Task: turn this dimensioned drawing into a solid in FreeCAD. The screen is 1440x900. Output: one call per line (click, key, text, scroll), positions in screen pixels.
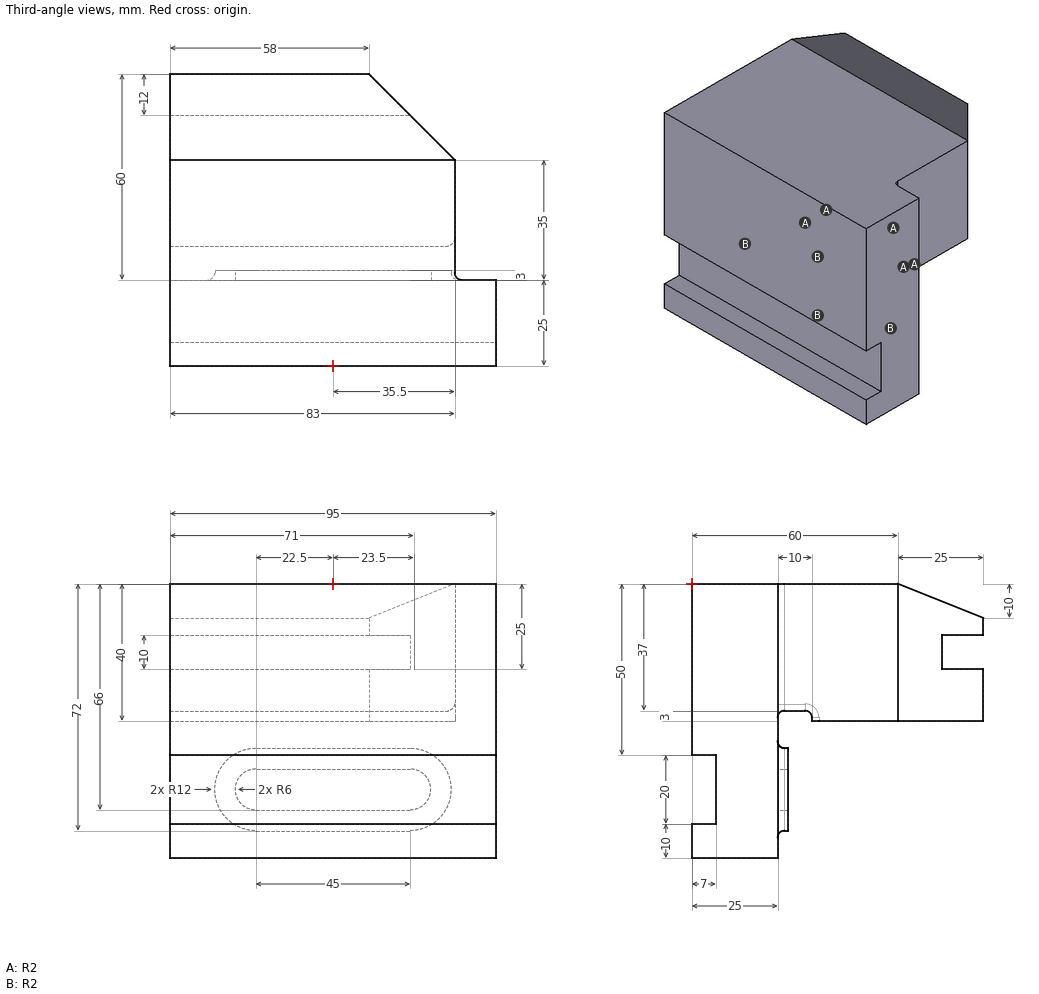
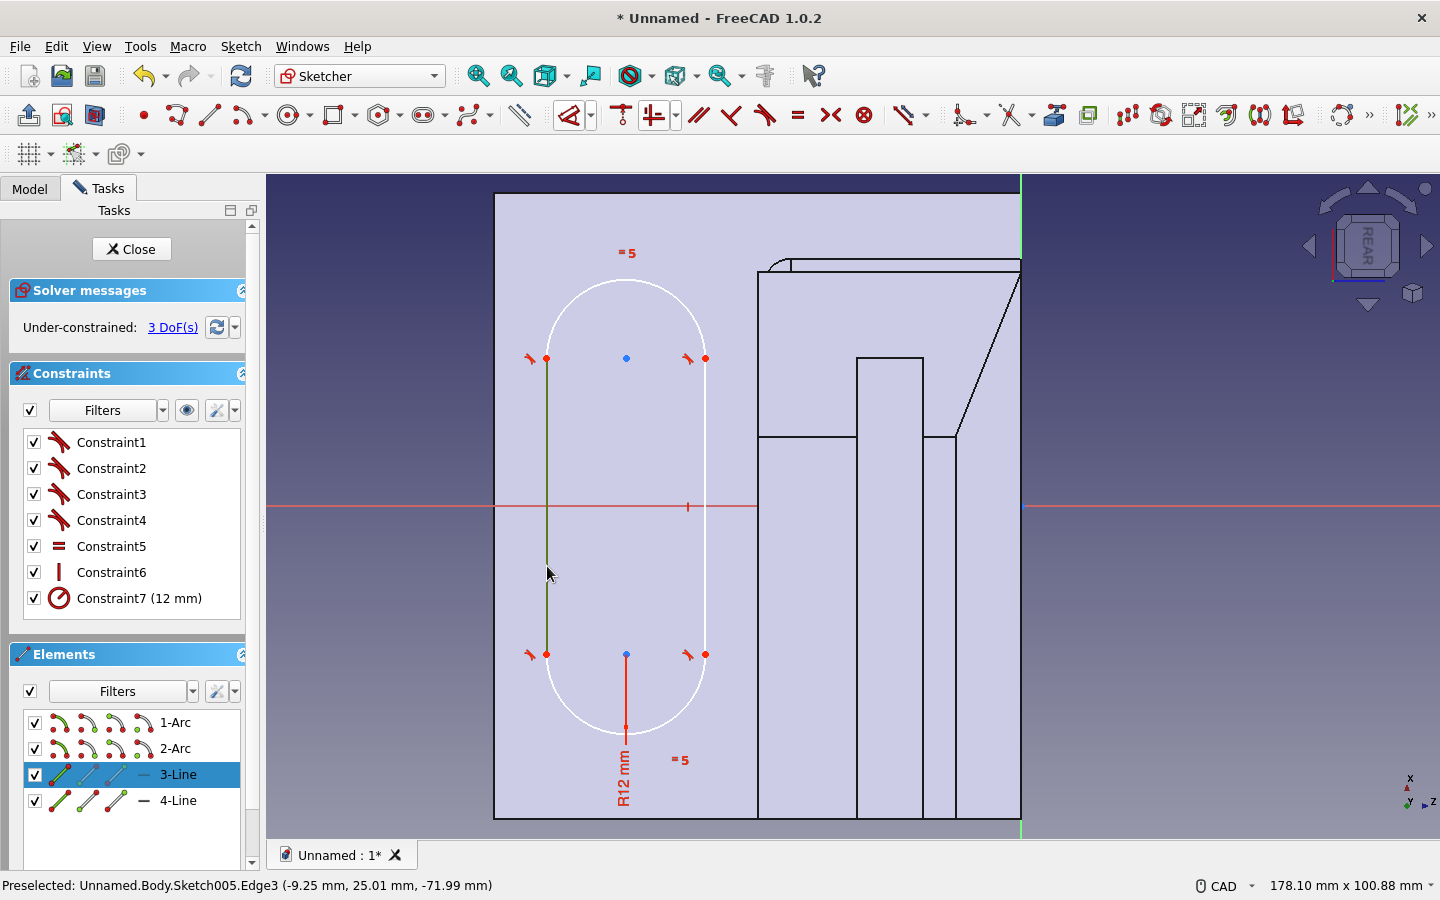
click(590, 116)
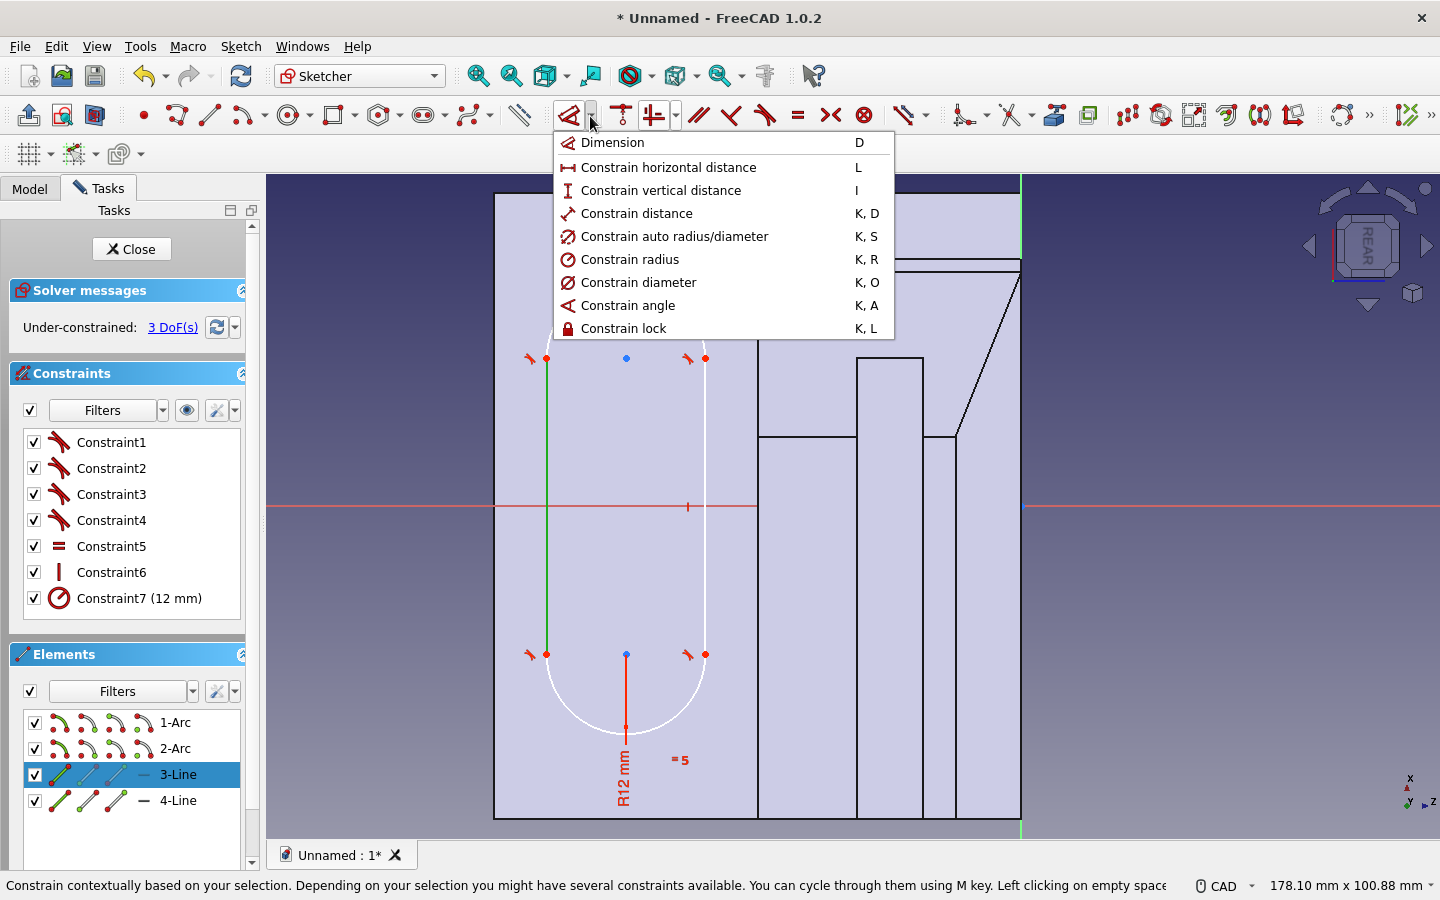
click(724, 190)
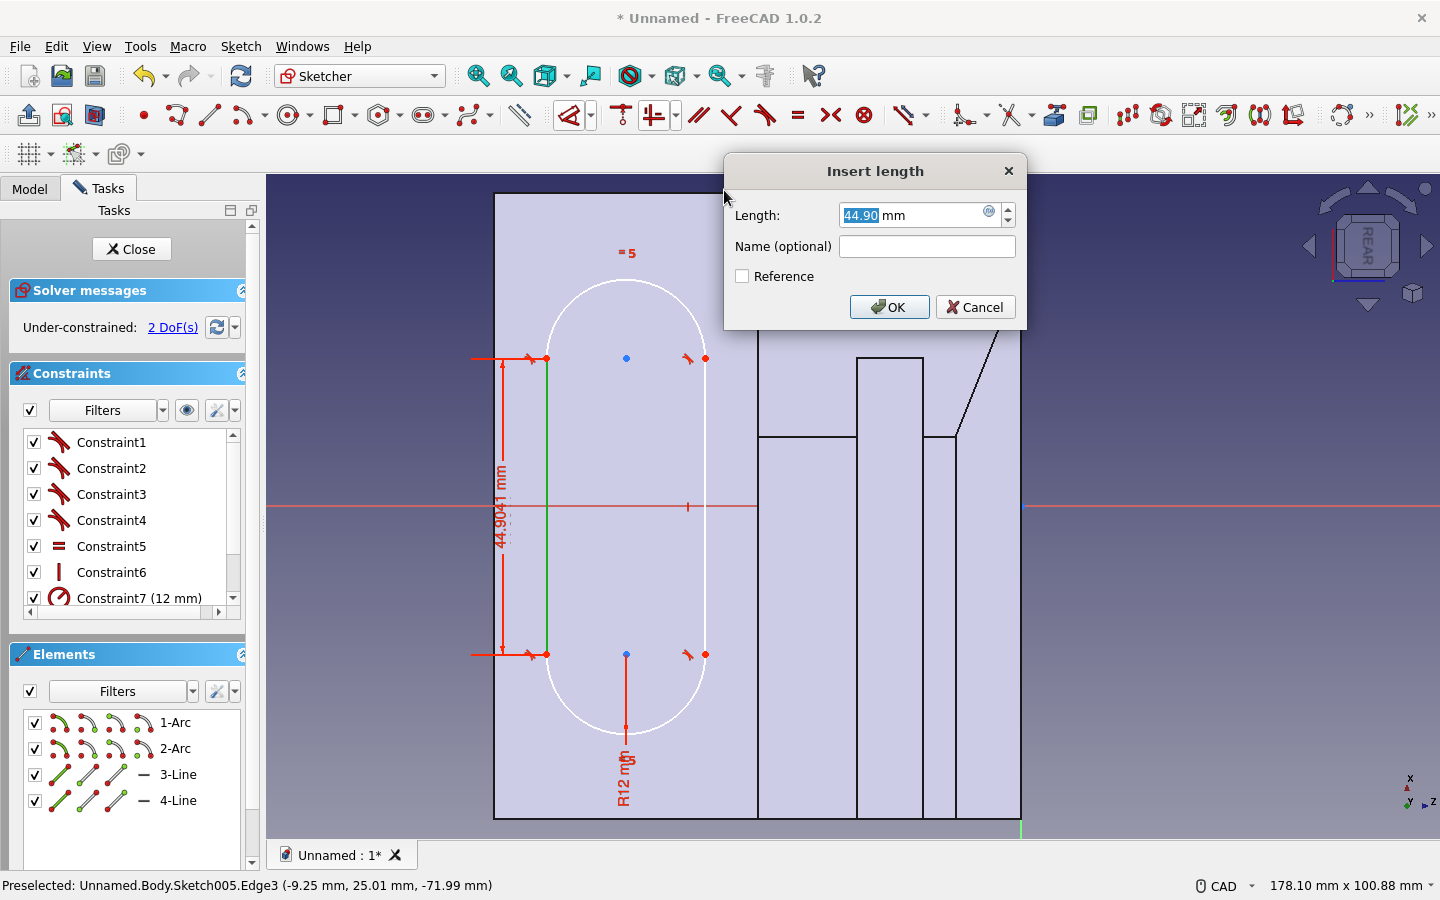
text(45)
key(Return)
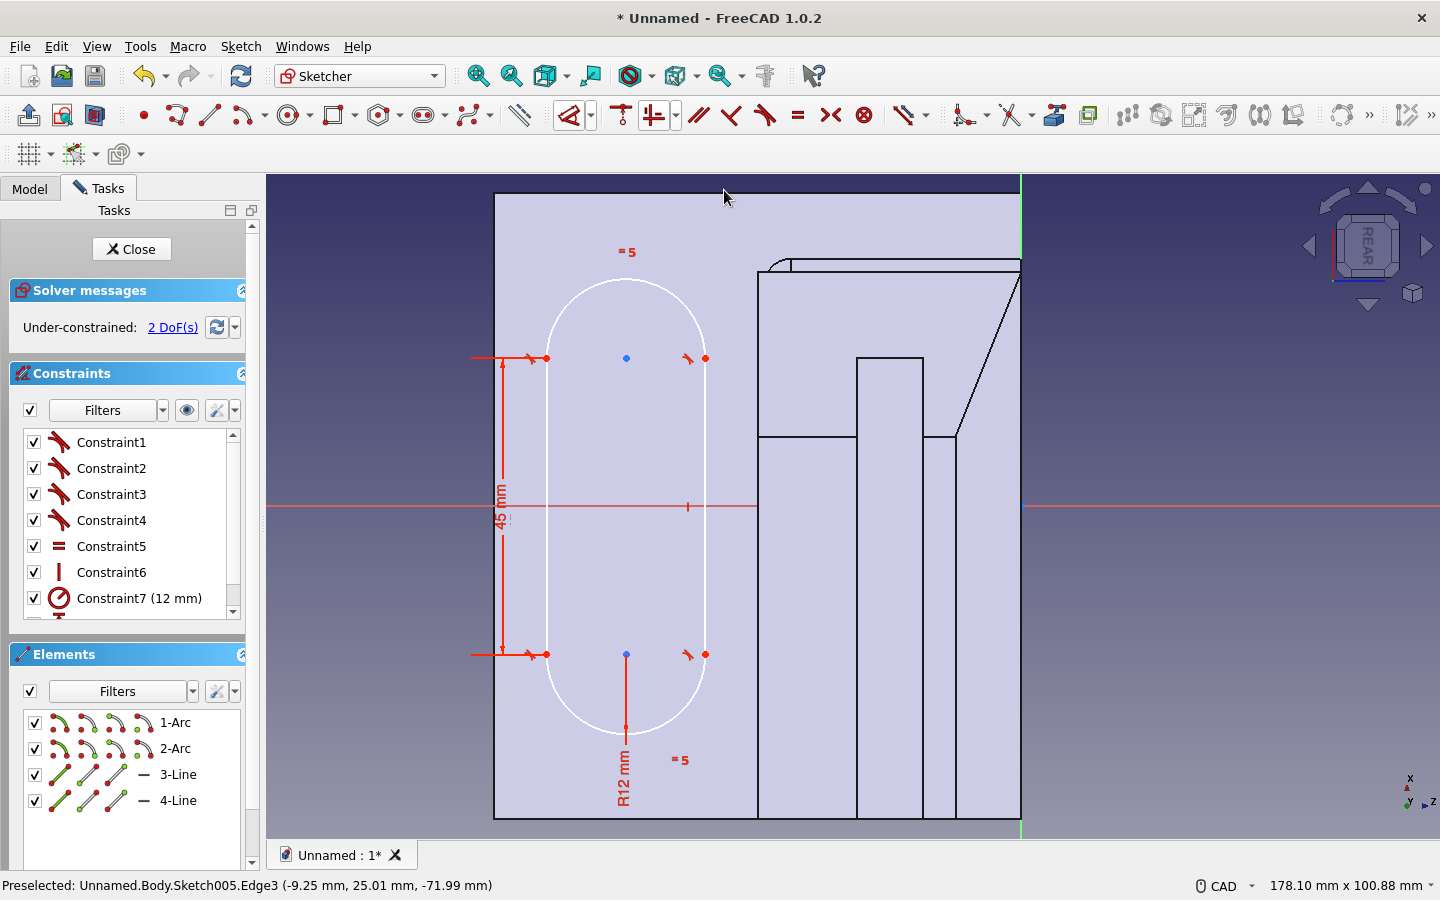
click(547, 655)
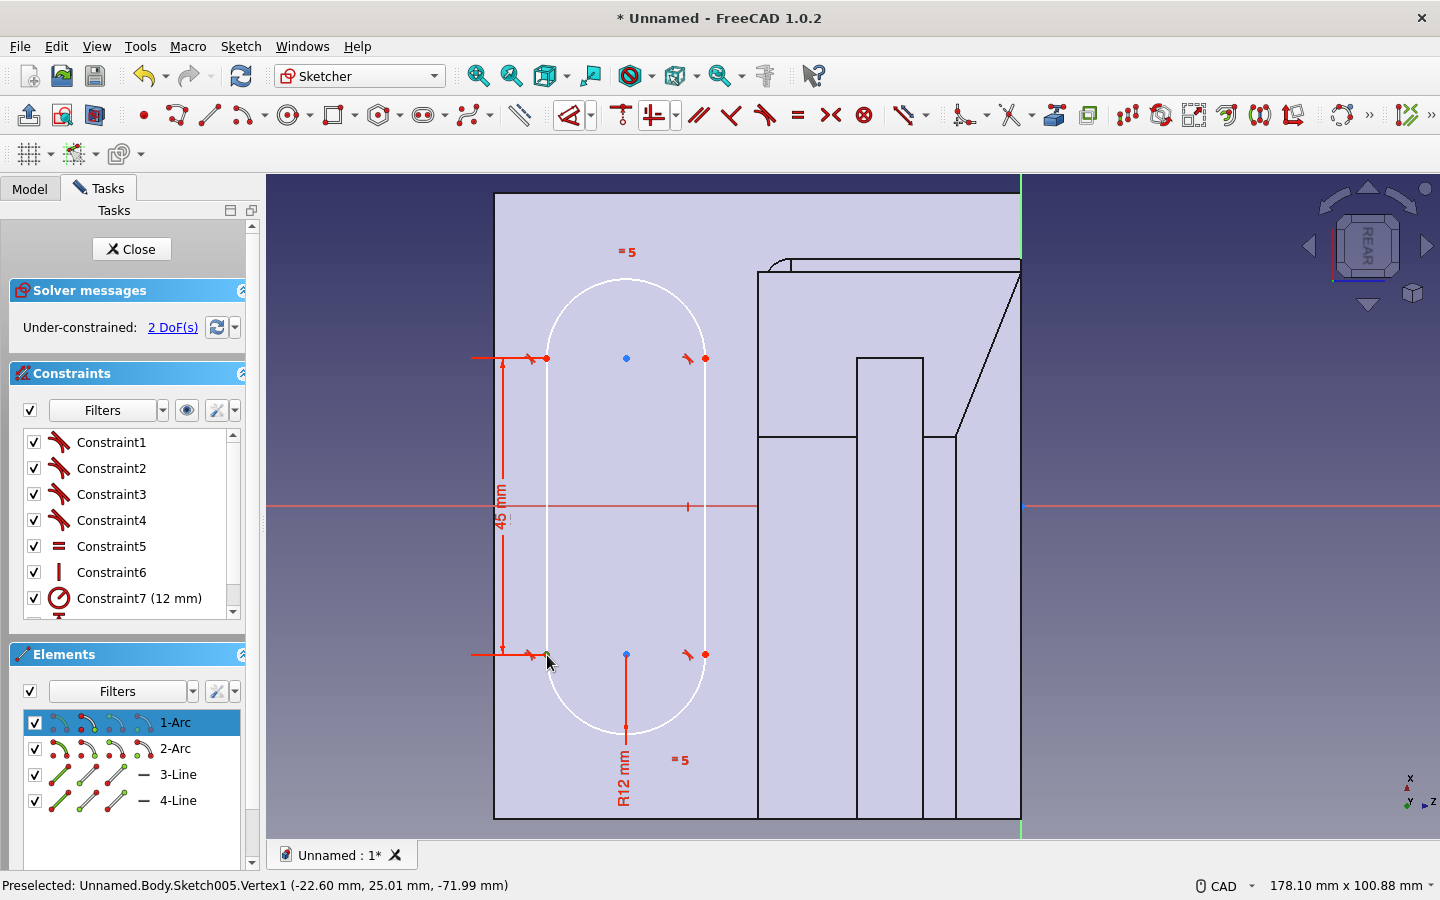
click(590, 116)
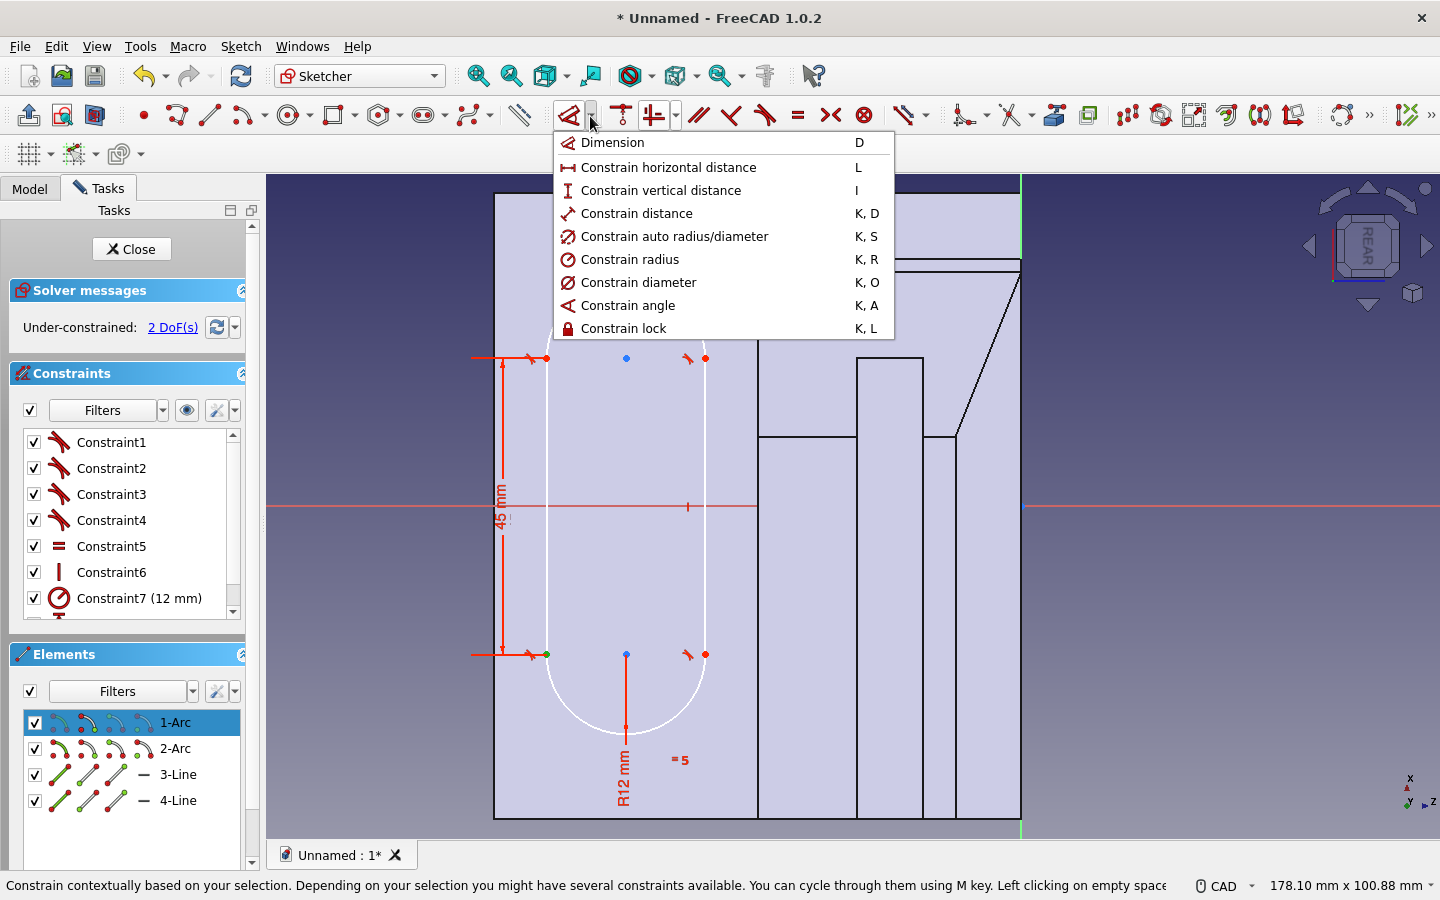
click(724, 168)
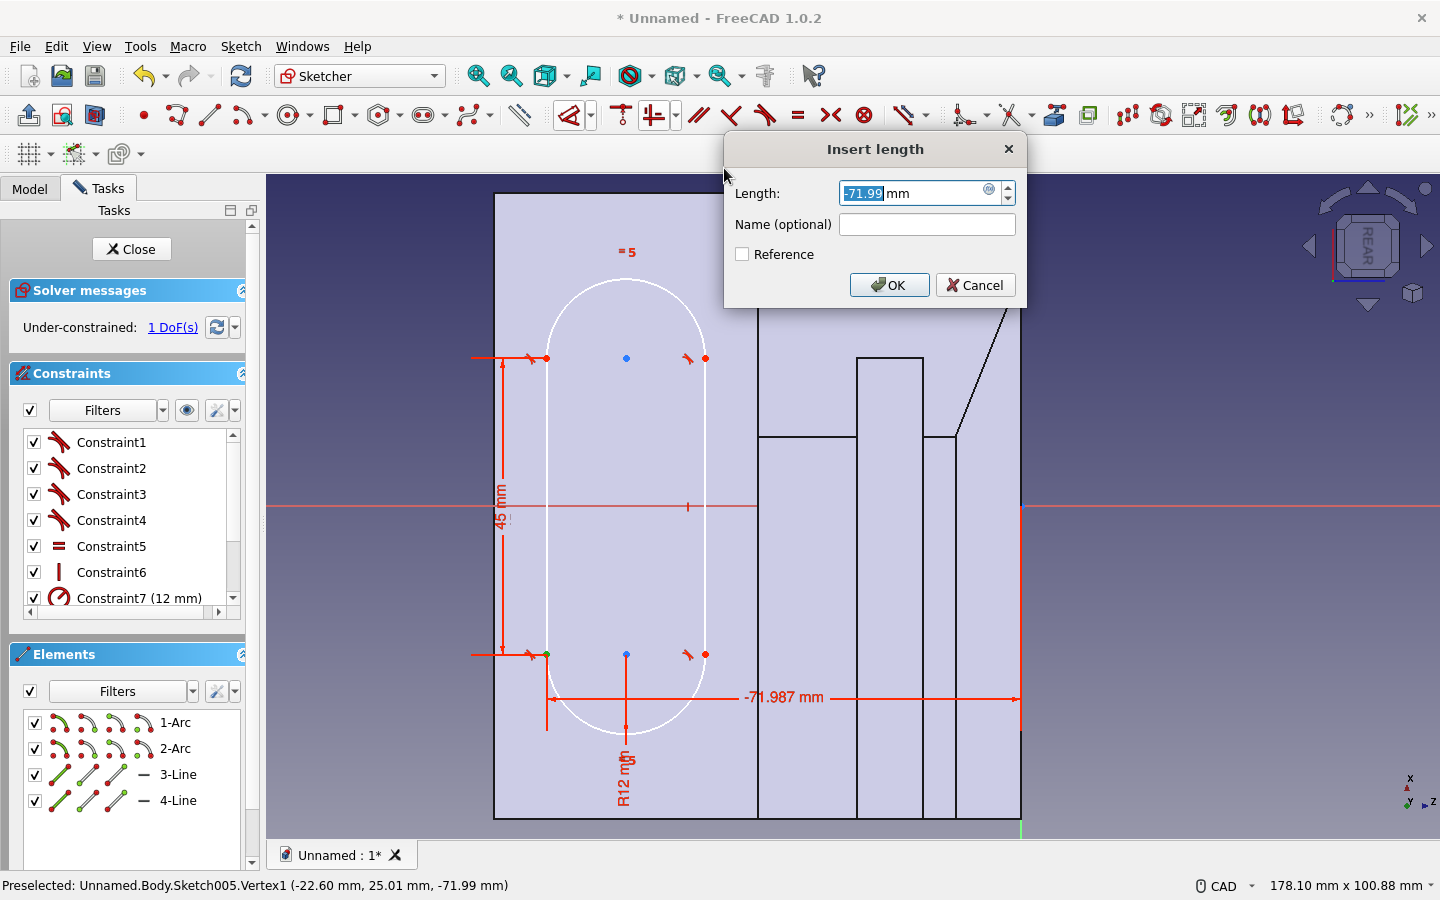
text(-72)
key(Return)